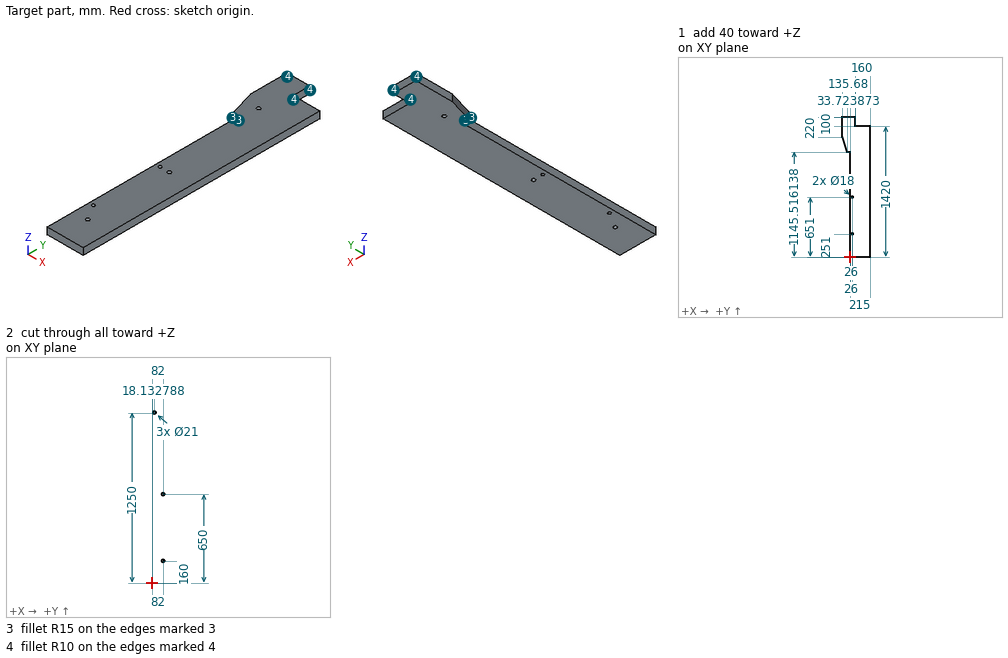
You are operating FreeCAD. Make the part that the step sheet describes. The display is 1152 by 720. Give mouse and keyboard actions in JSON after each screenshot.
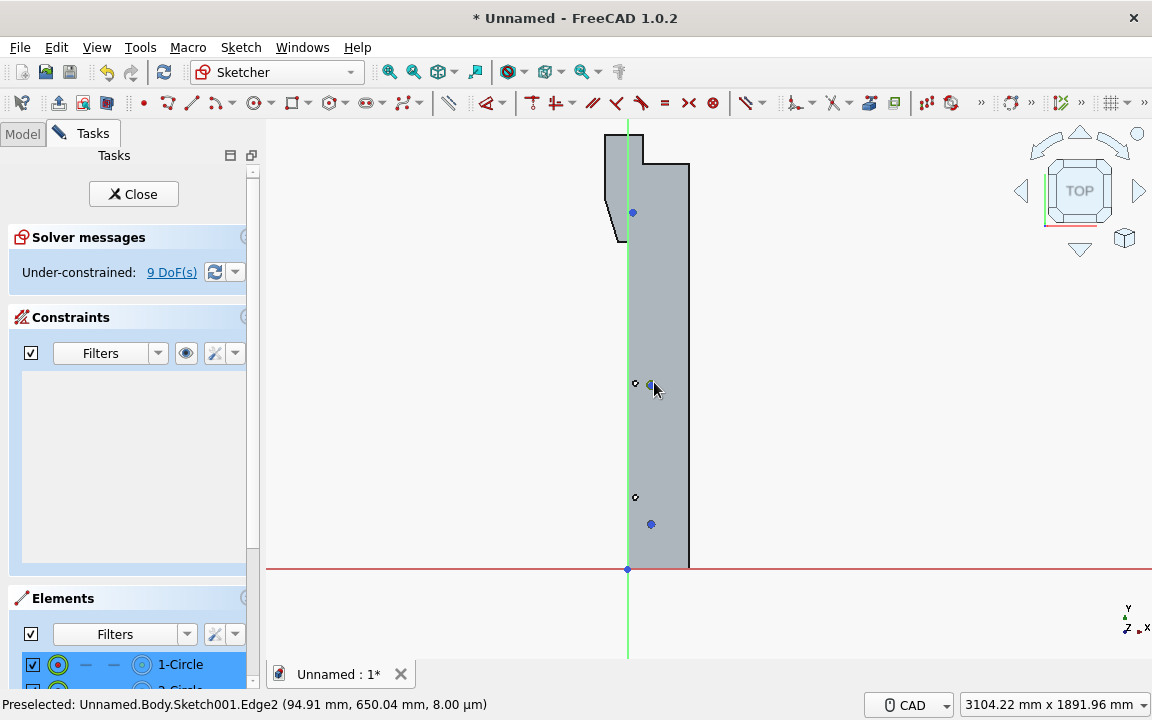
{"action": "scroll", "coordinate": [653, 522], "scroll_direction": "up", "scroll_amount": 7}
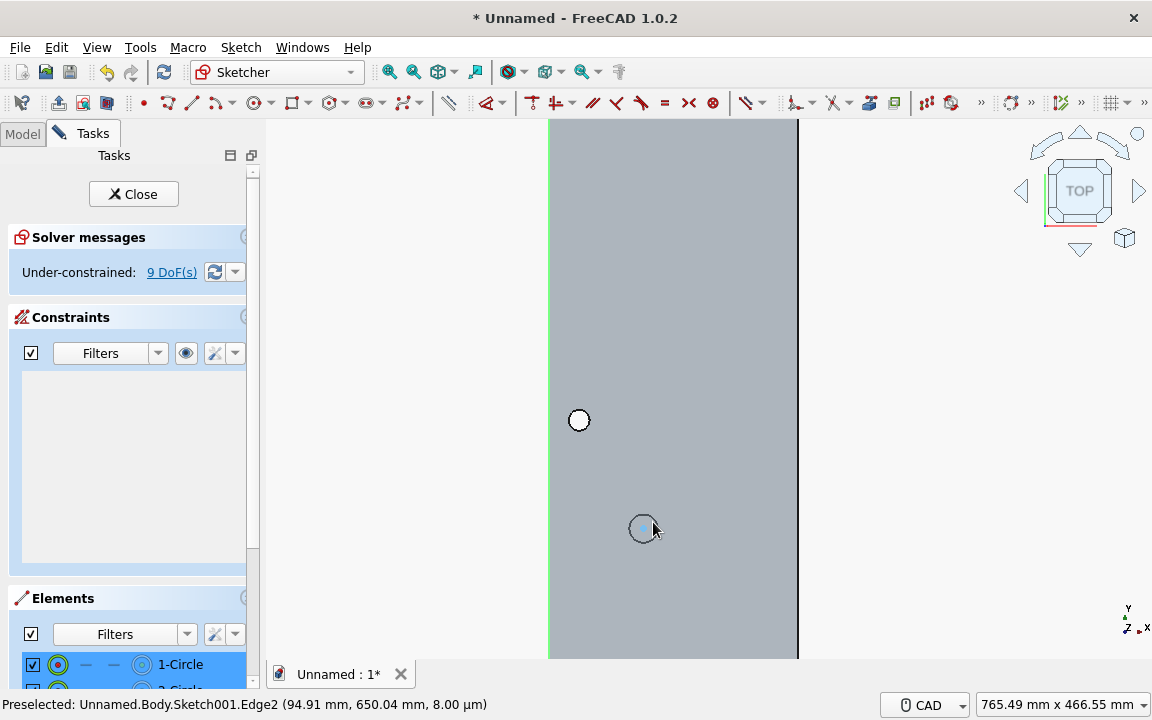
{"action": "left_click", "coordinate": [654, 519]}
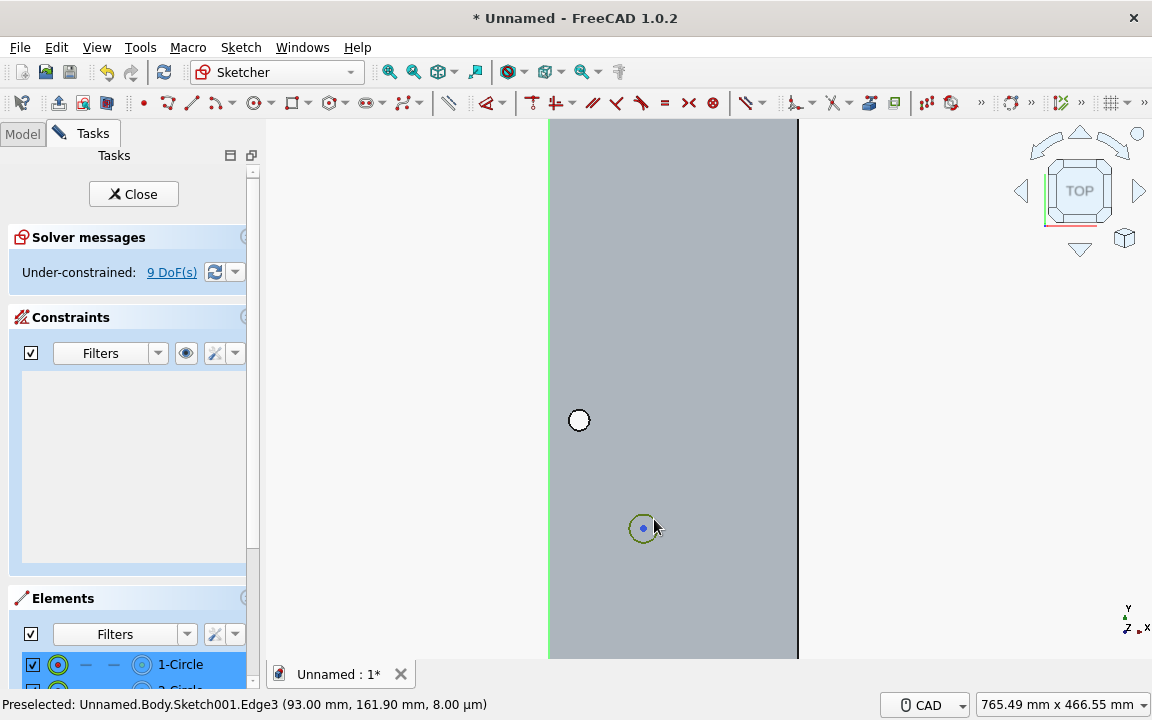
{"action": "key", "text": "e"}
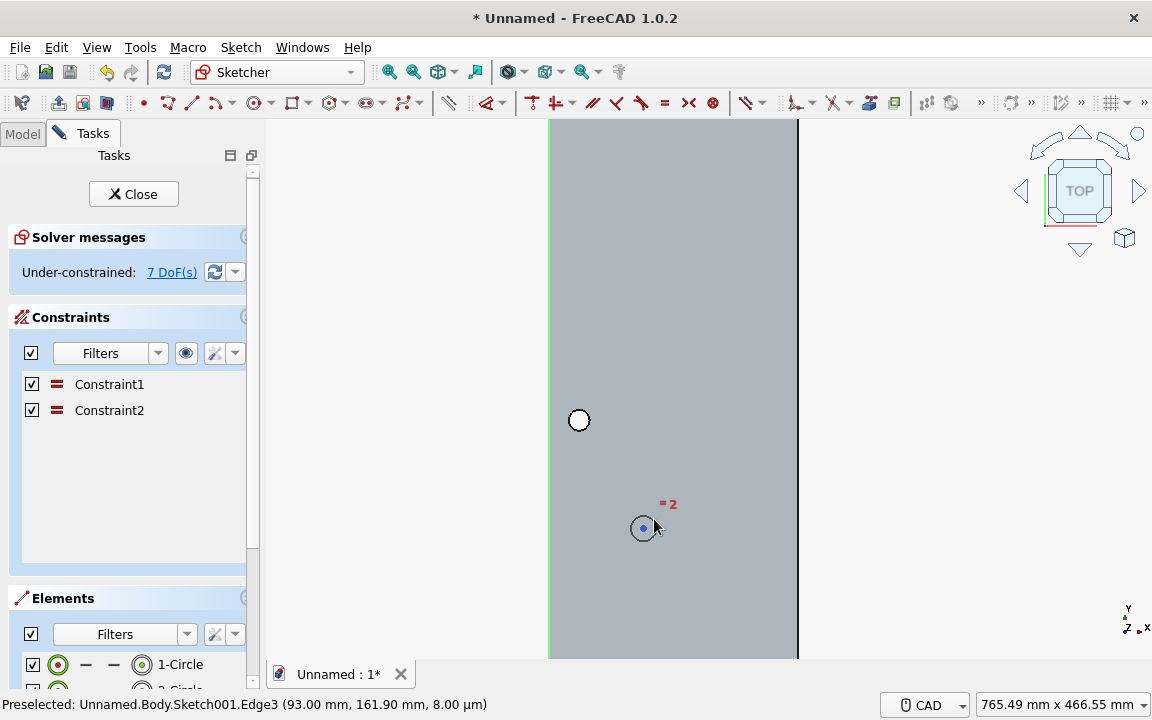
{"action": "key", "text": "d"}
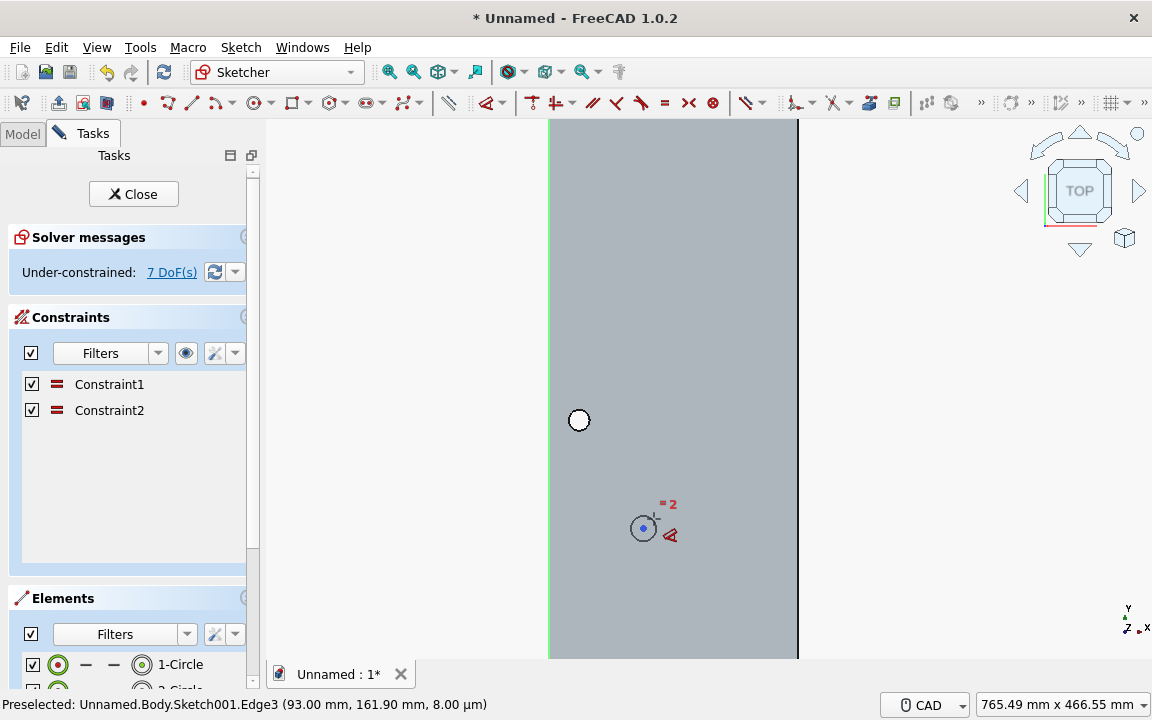
{"action": "scroll", "coordinate": [653, 522], "scroll_direction": "down", "scroll_amount": 7}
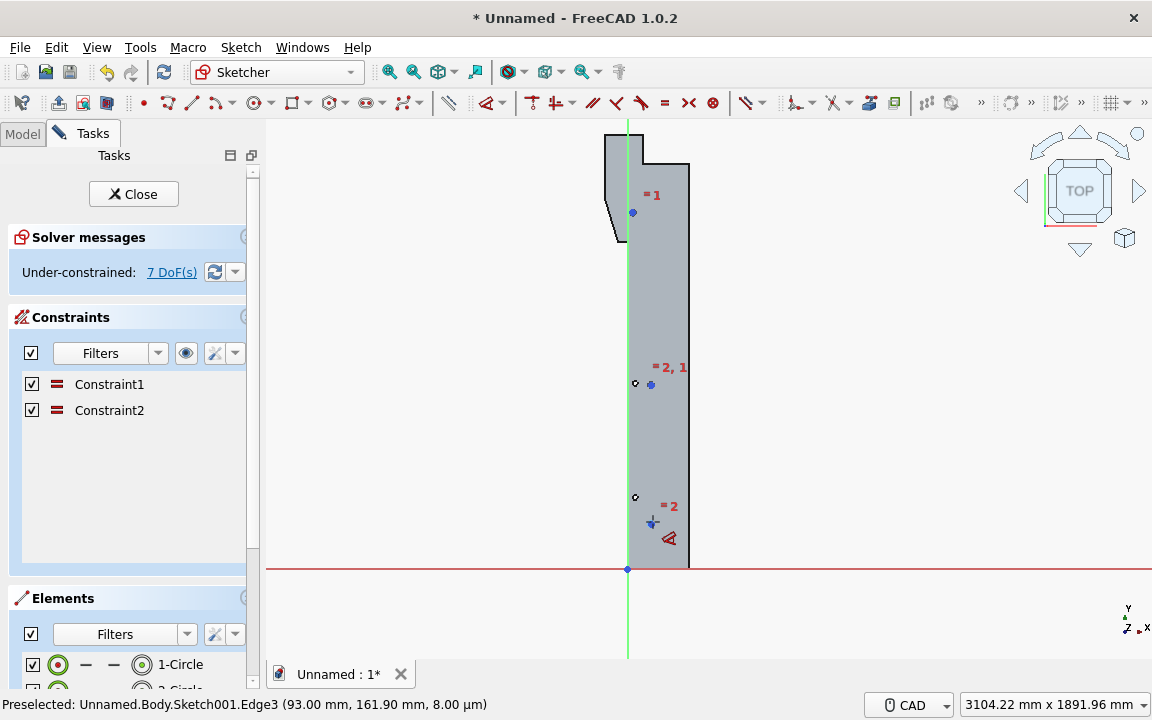
{"action": "scroll", "coordinate": [635, 210], "scroll_direction": "up", "scroll_amount": 10}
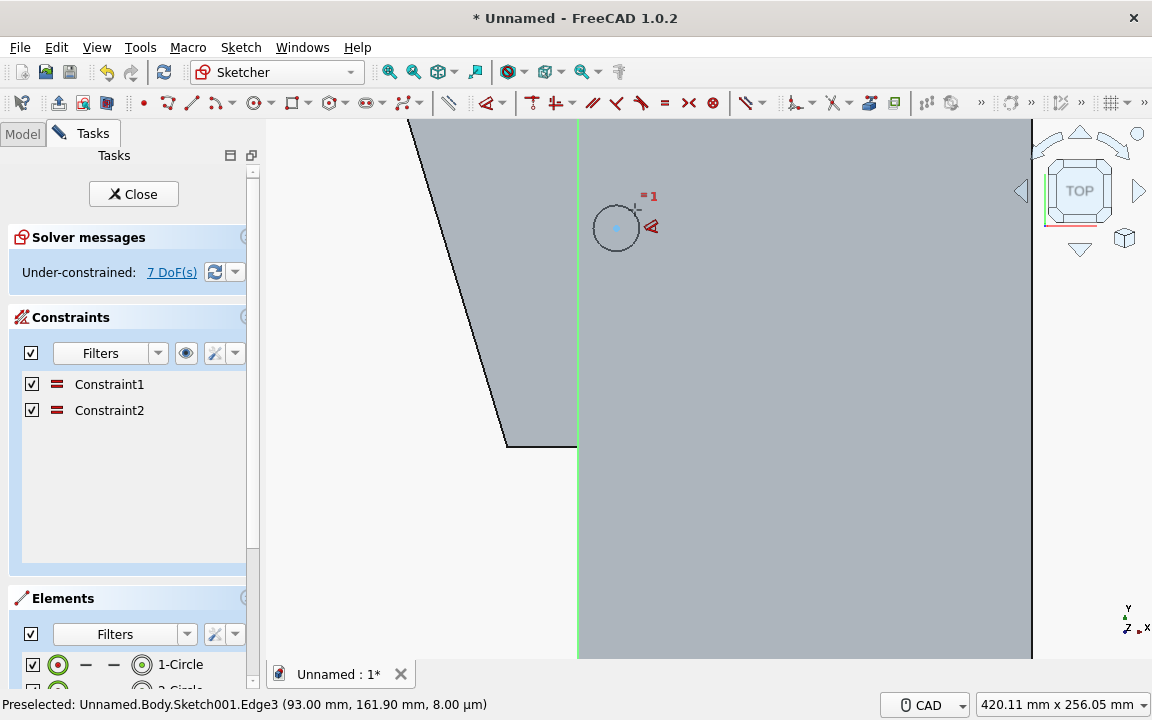
{"action": "left_click", "coordinate": [633, 212]}
{"action": "left_click", "coordinate": [656, 190]}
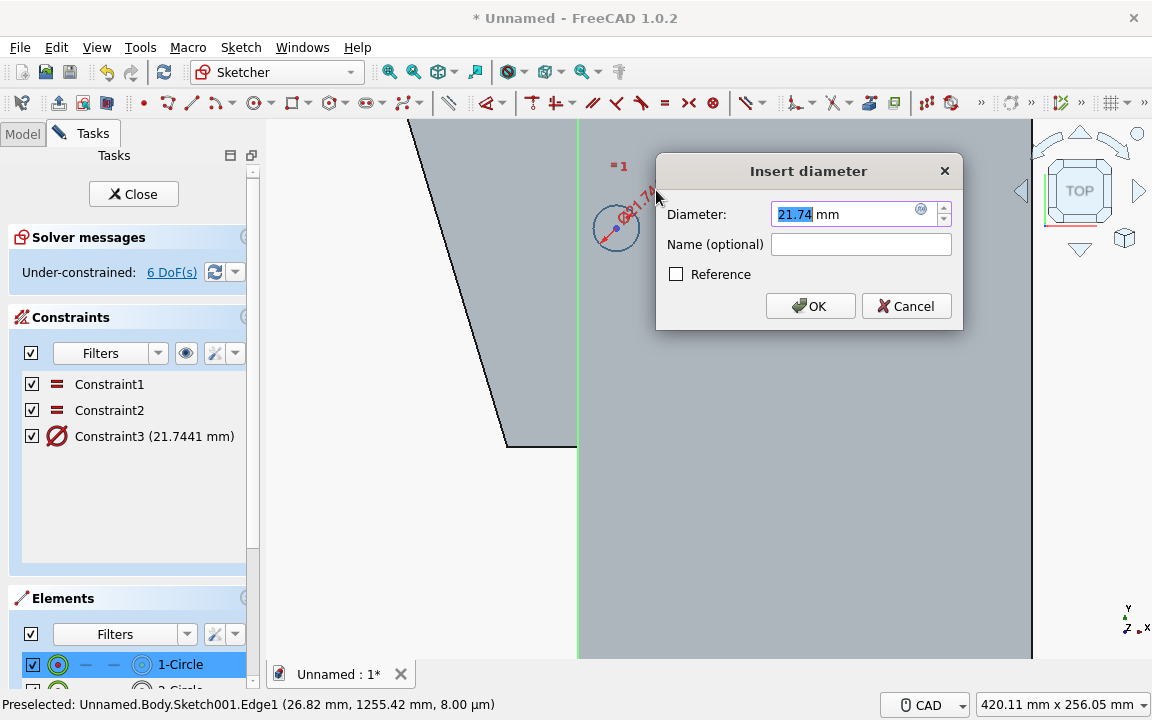
{"action": "type", "text": "21"}
{"action": "key", "text": "Return"}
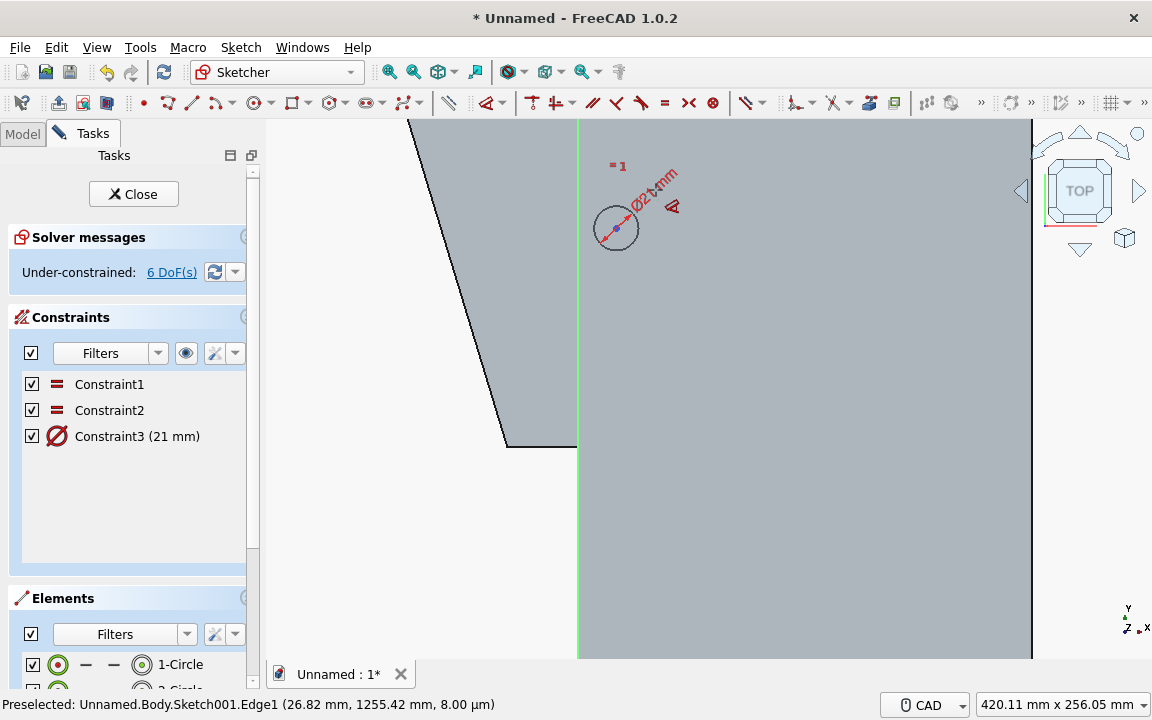
{"action": "scroll", "coordinate": [635, 210], "scroll_direction": "down", "scroll_amount": 10}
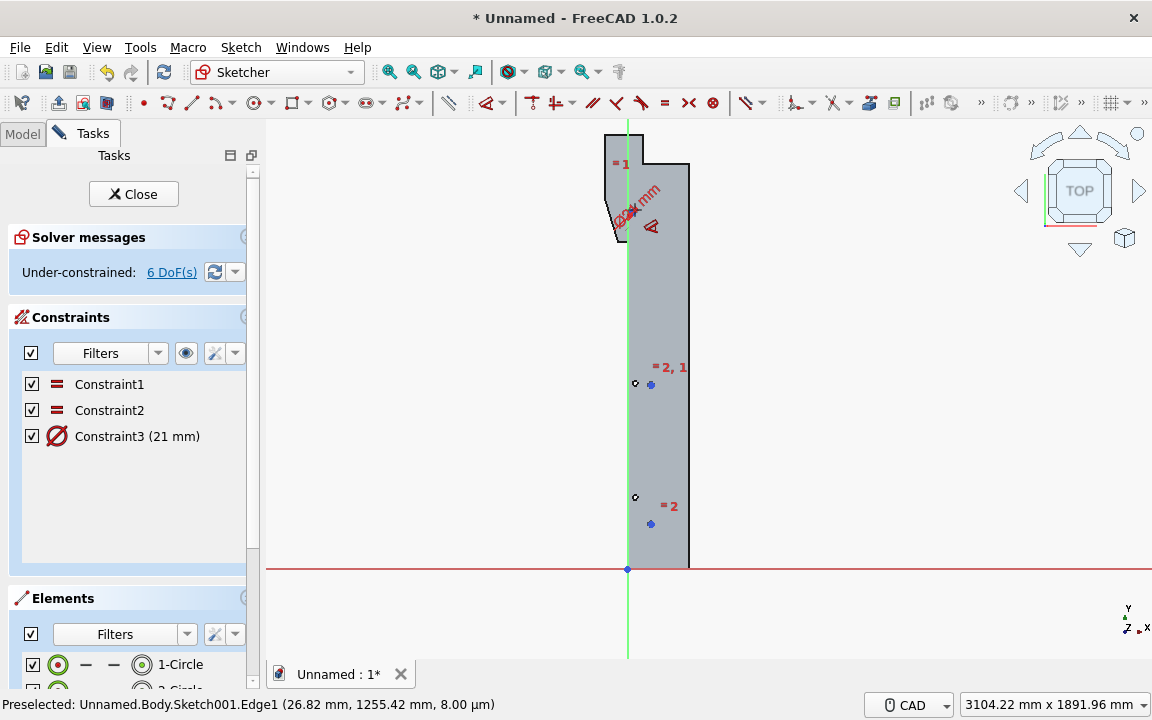
{"action": "scroll", "coordinate": [651, 385], "scroll_direction": "up", "scroll_amount": 3}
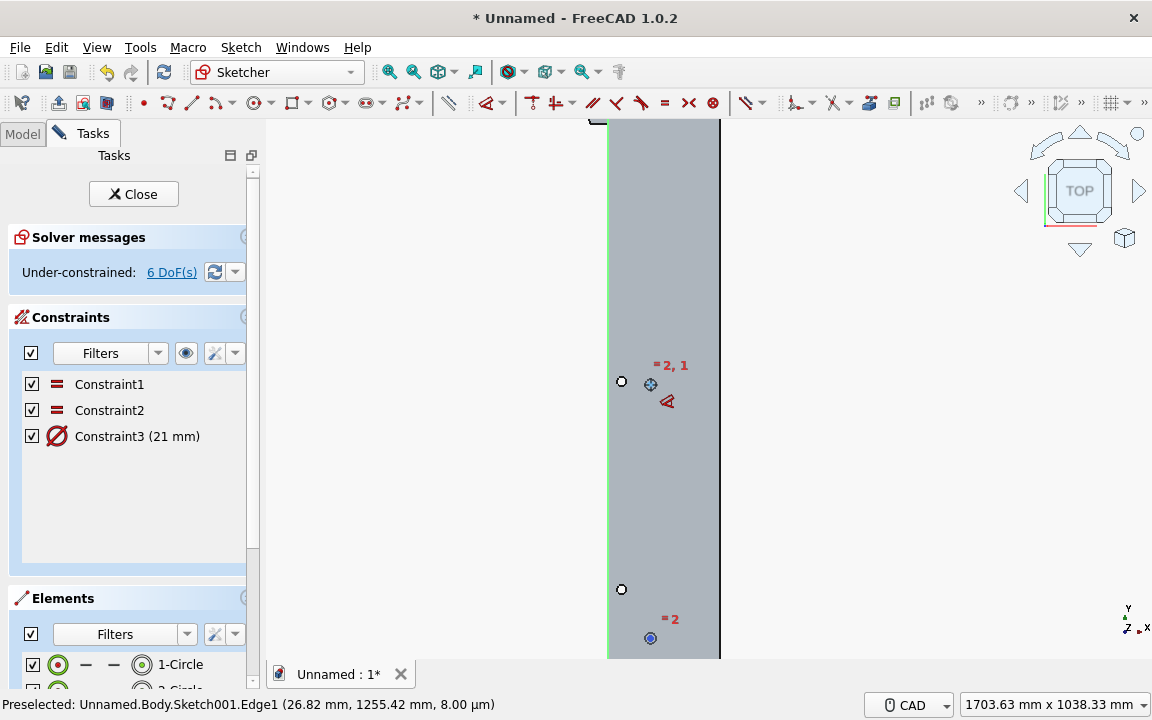
{"action": "left_click", "coordinate": [651, 385]}
{"action": "left_click", "coordinate": [629, 351]}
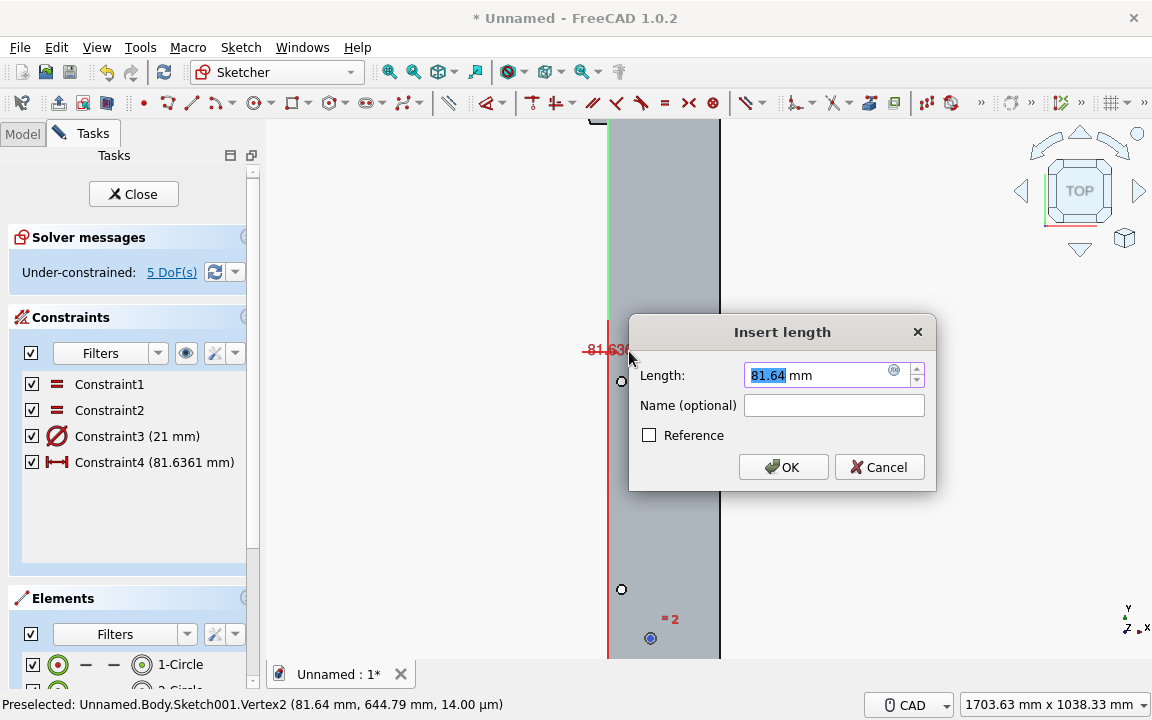
{"action": "type", "text": "82"}
{"action": "key", "text": "Return"}